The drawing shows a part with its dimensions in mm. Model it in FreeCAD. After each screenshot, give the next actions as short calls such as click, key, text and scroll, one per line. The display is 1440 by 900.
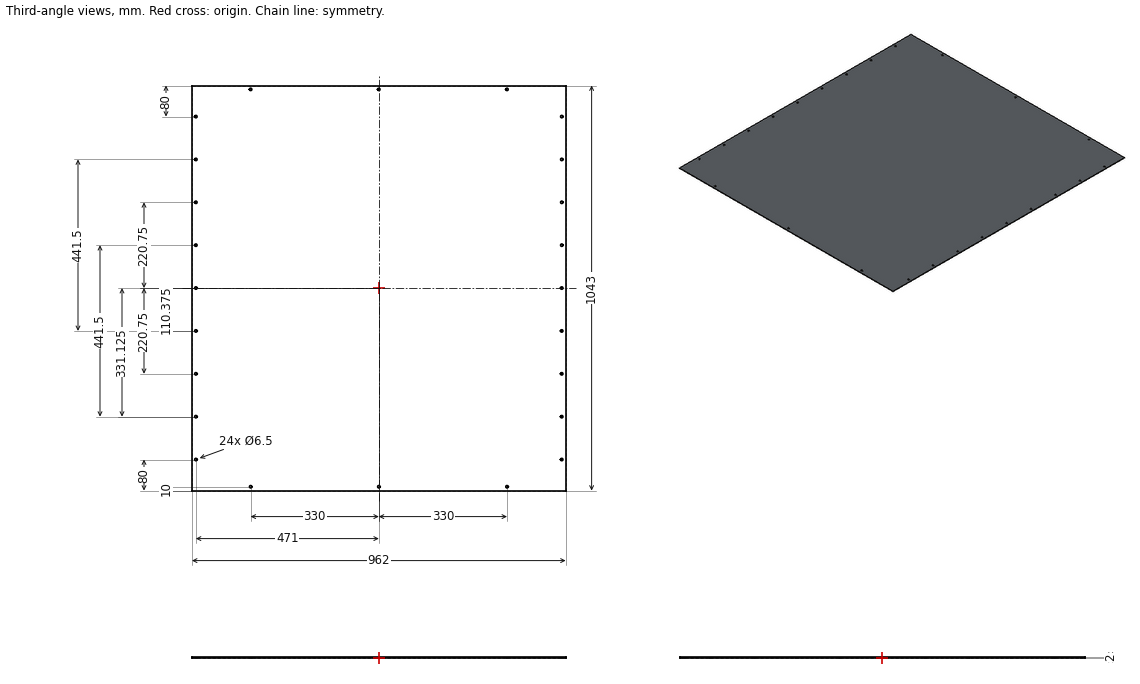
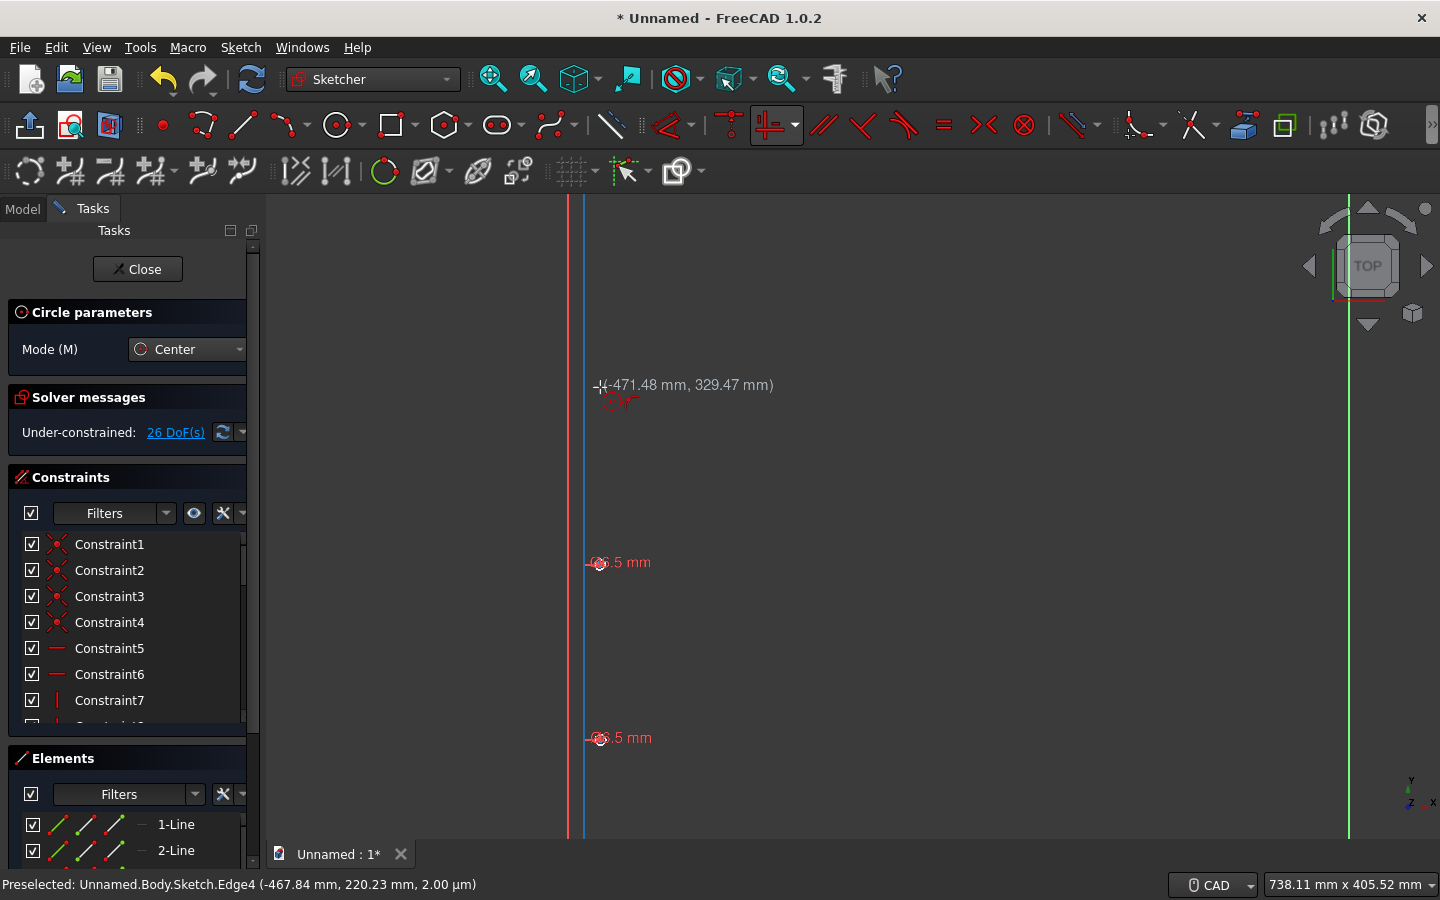
click(600, 388)
move(604, 384)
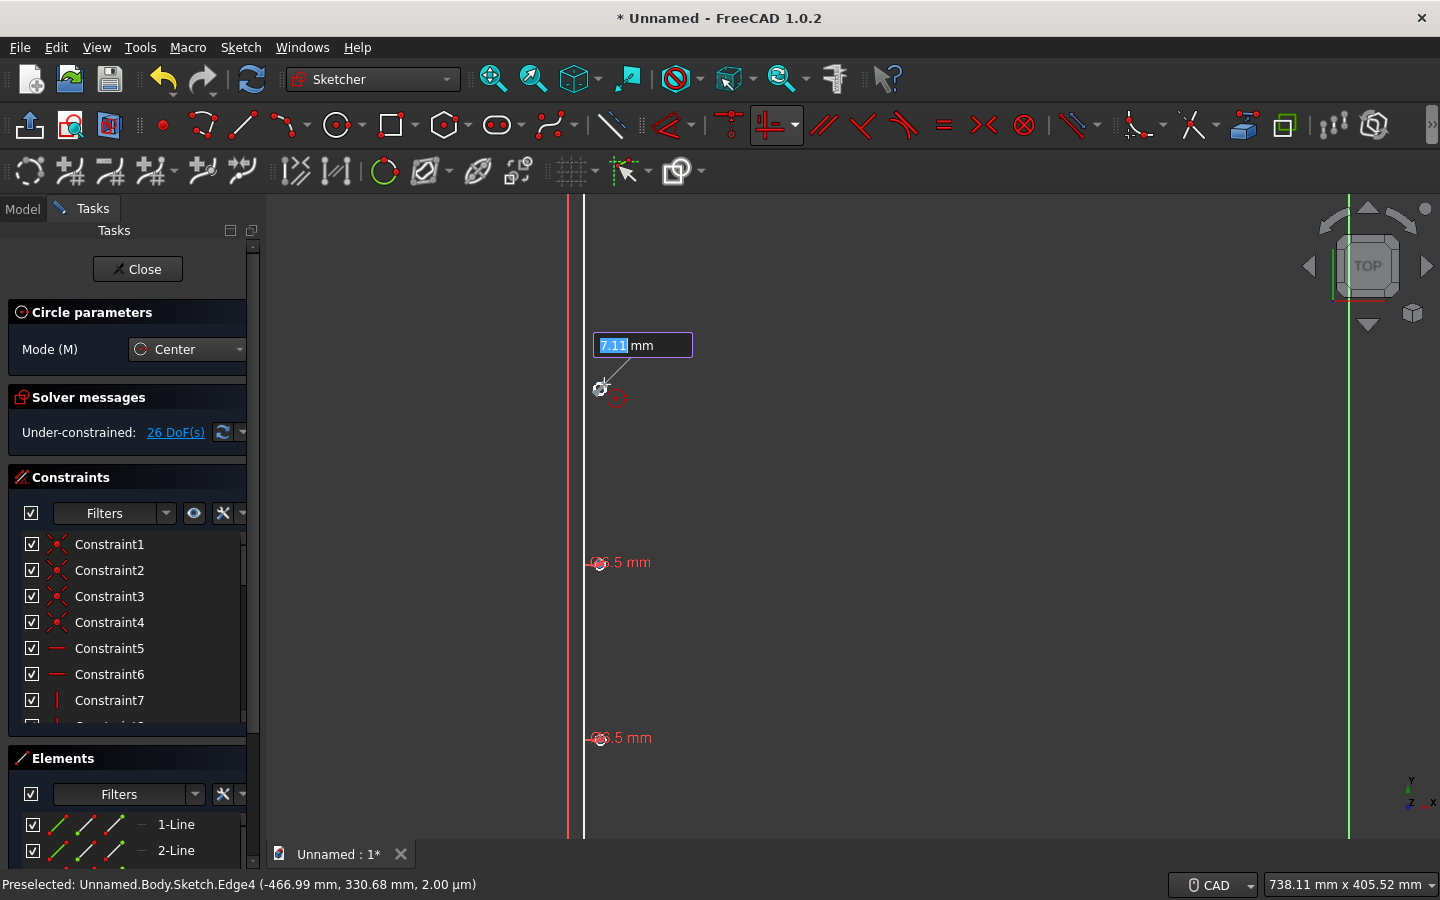
text(6.5)
key(Return)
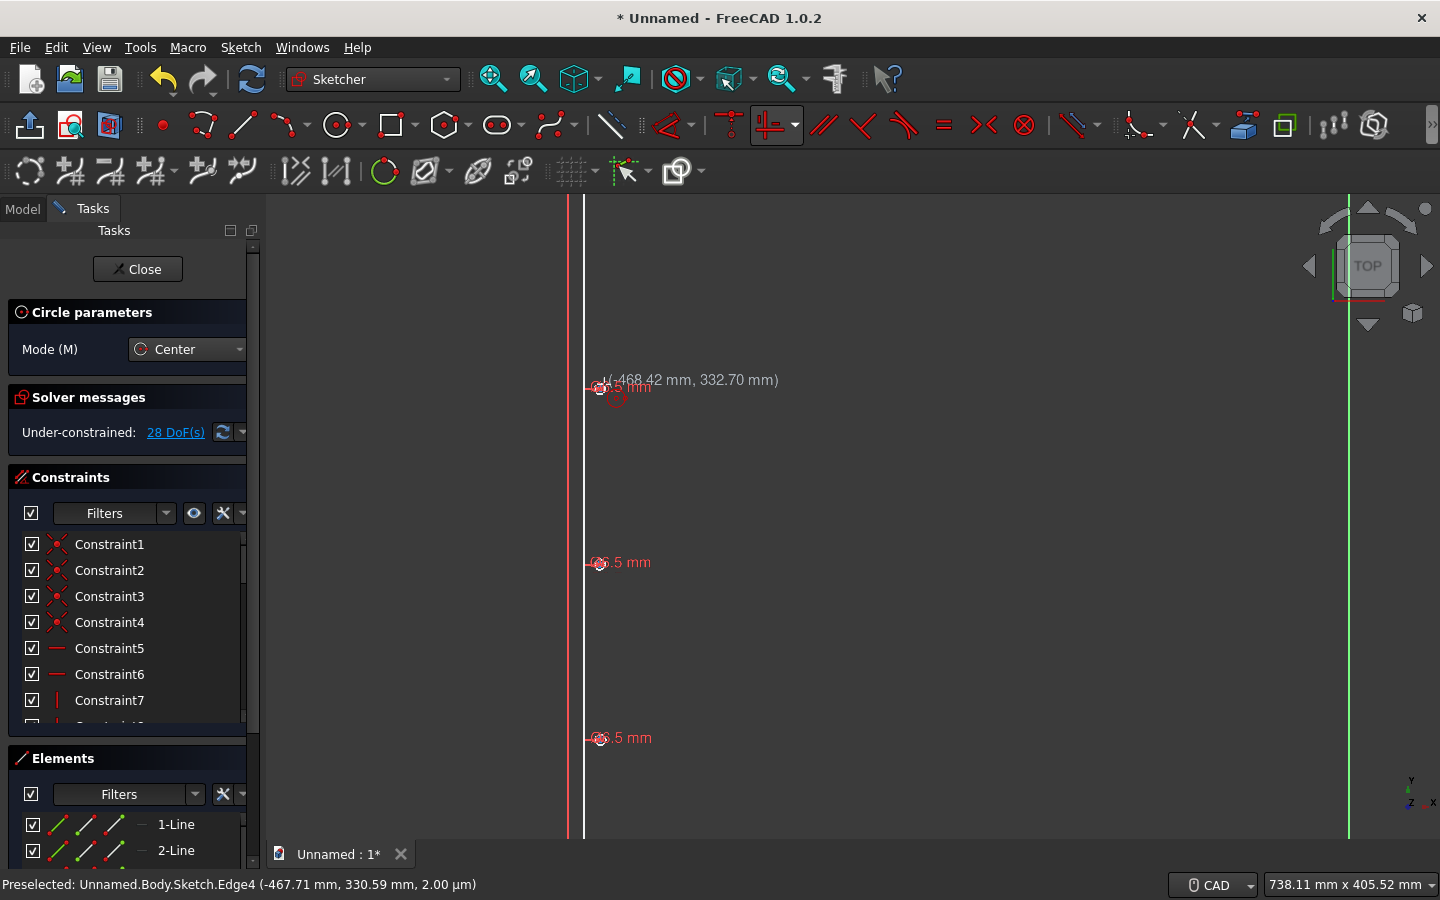
scroll(600, 386, down, 7)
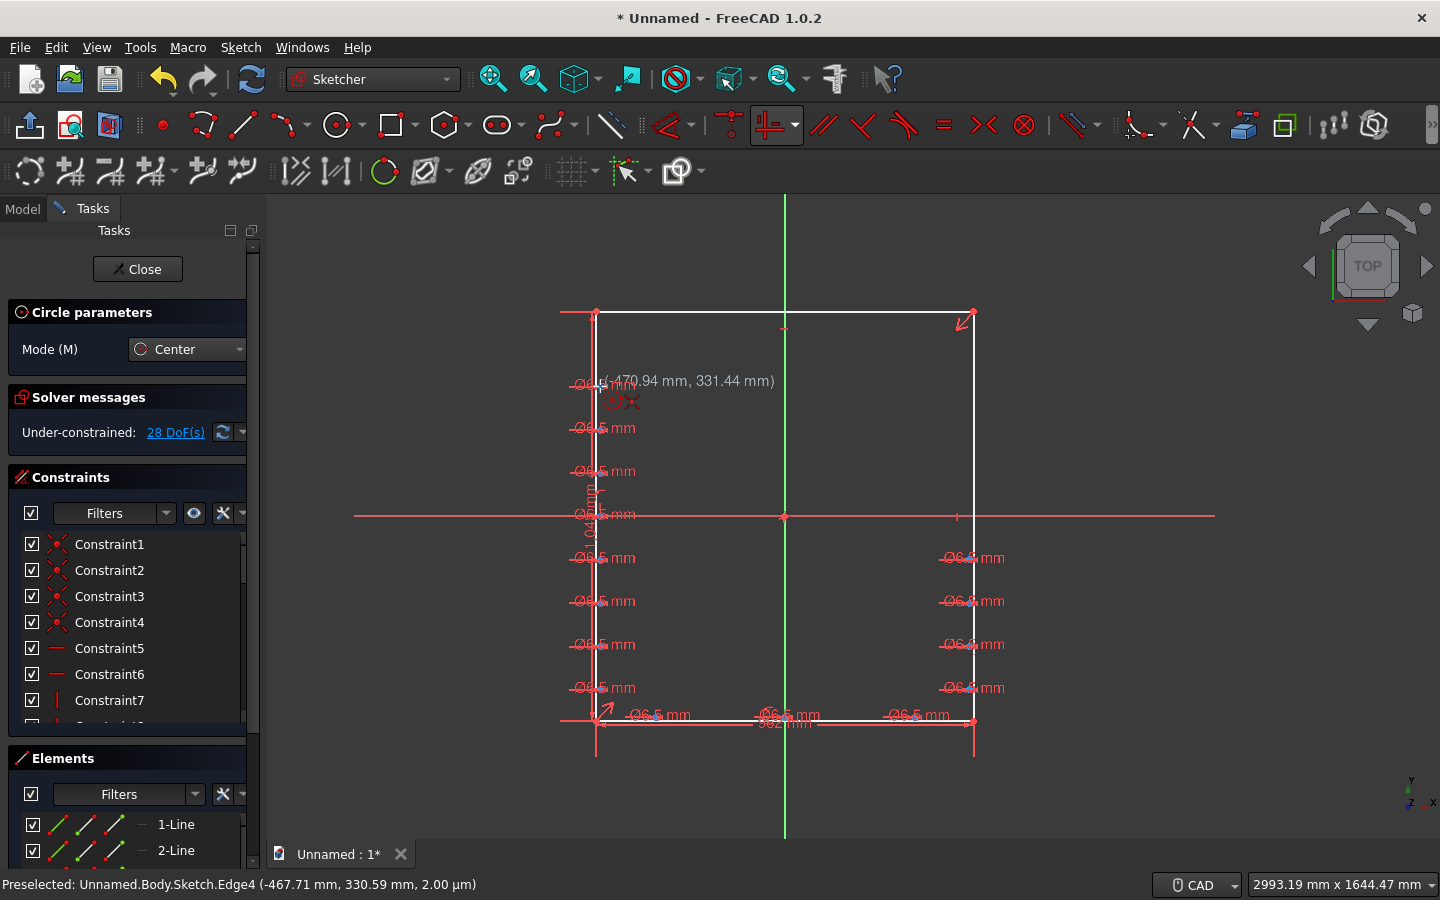
scroll(600, 343, up, 15)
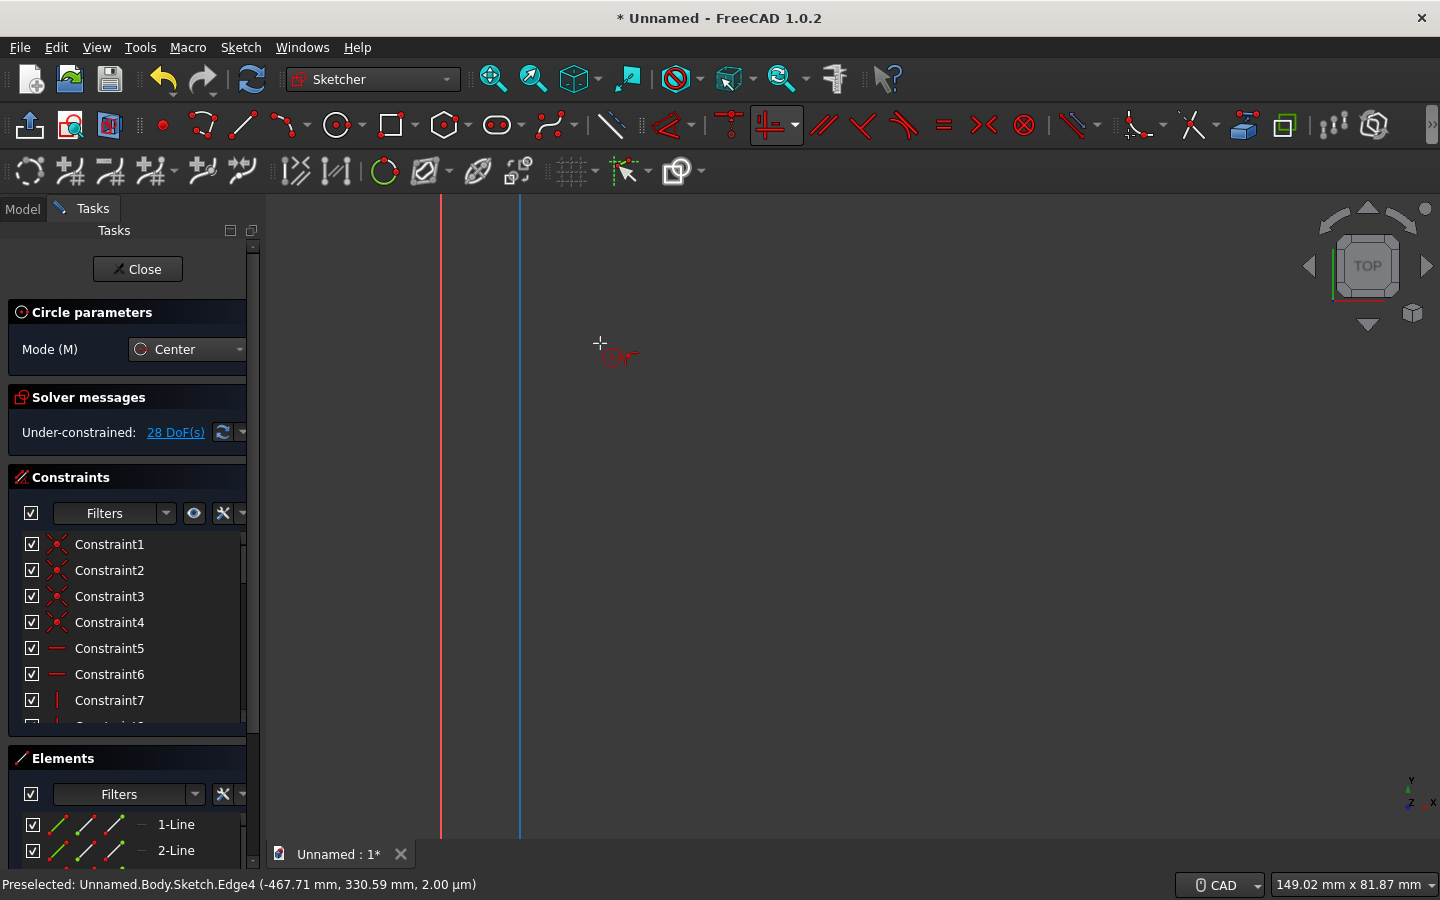
scroll(600, 343, down, 15)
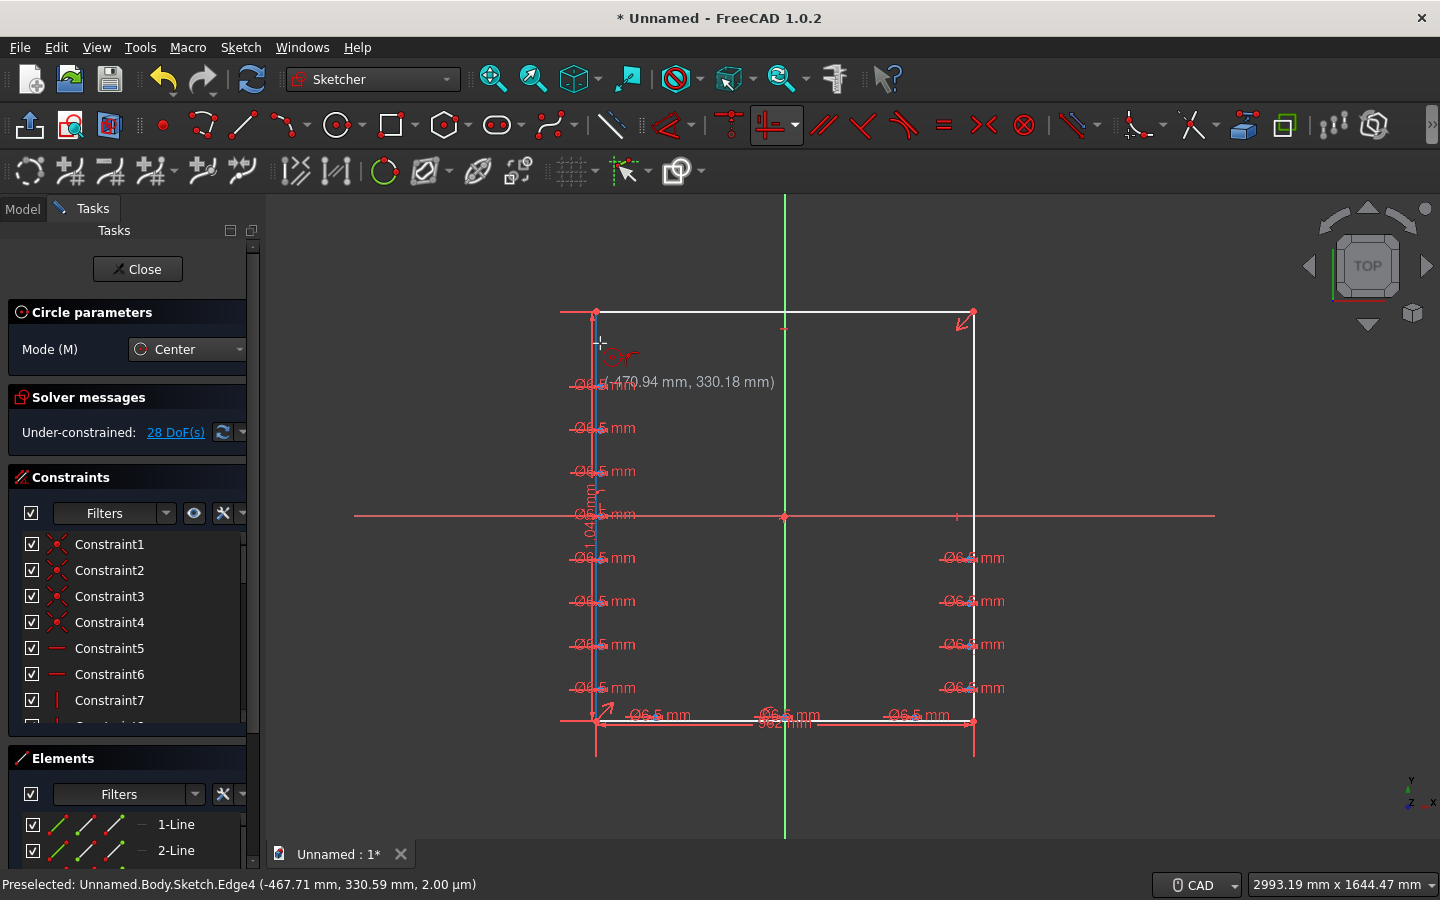
scroll(600, 343, up, 7)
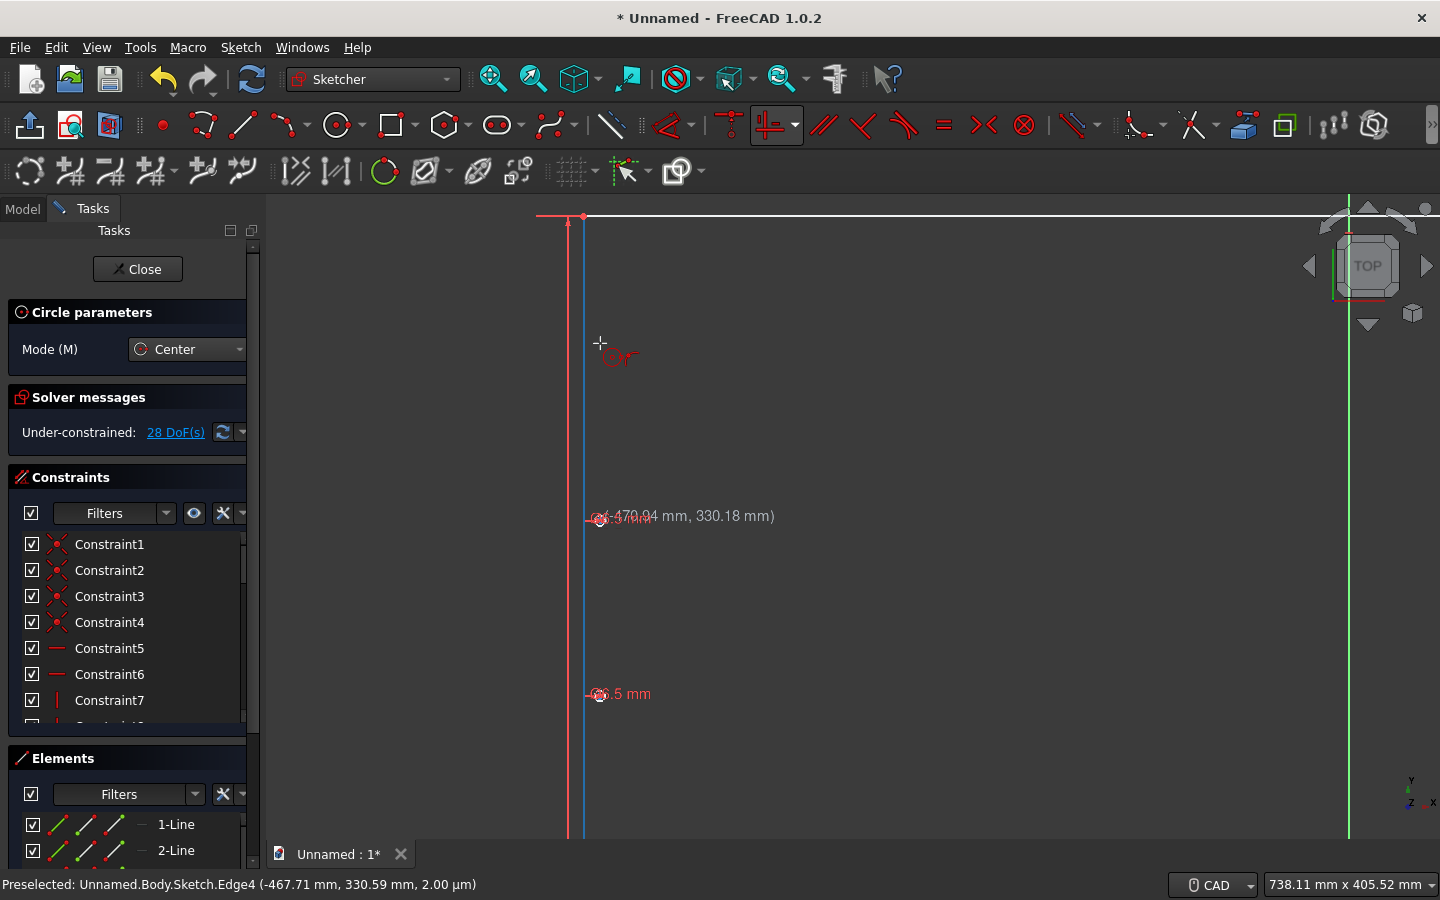
click(600, 344)
move(604, 340)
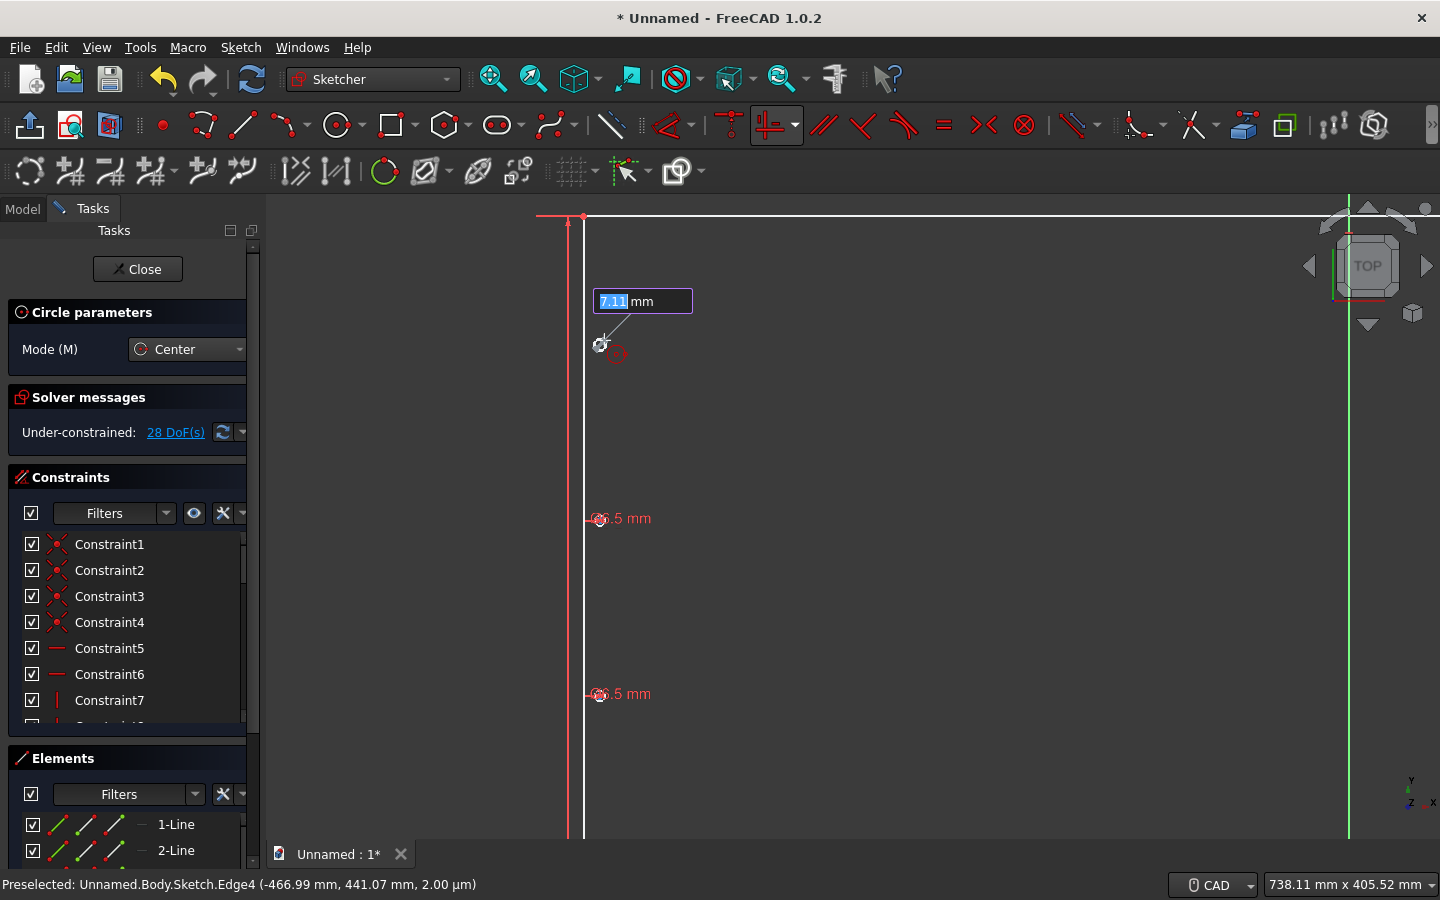
text(6.5)
key(Return)